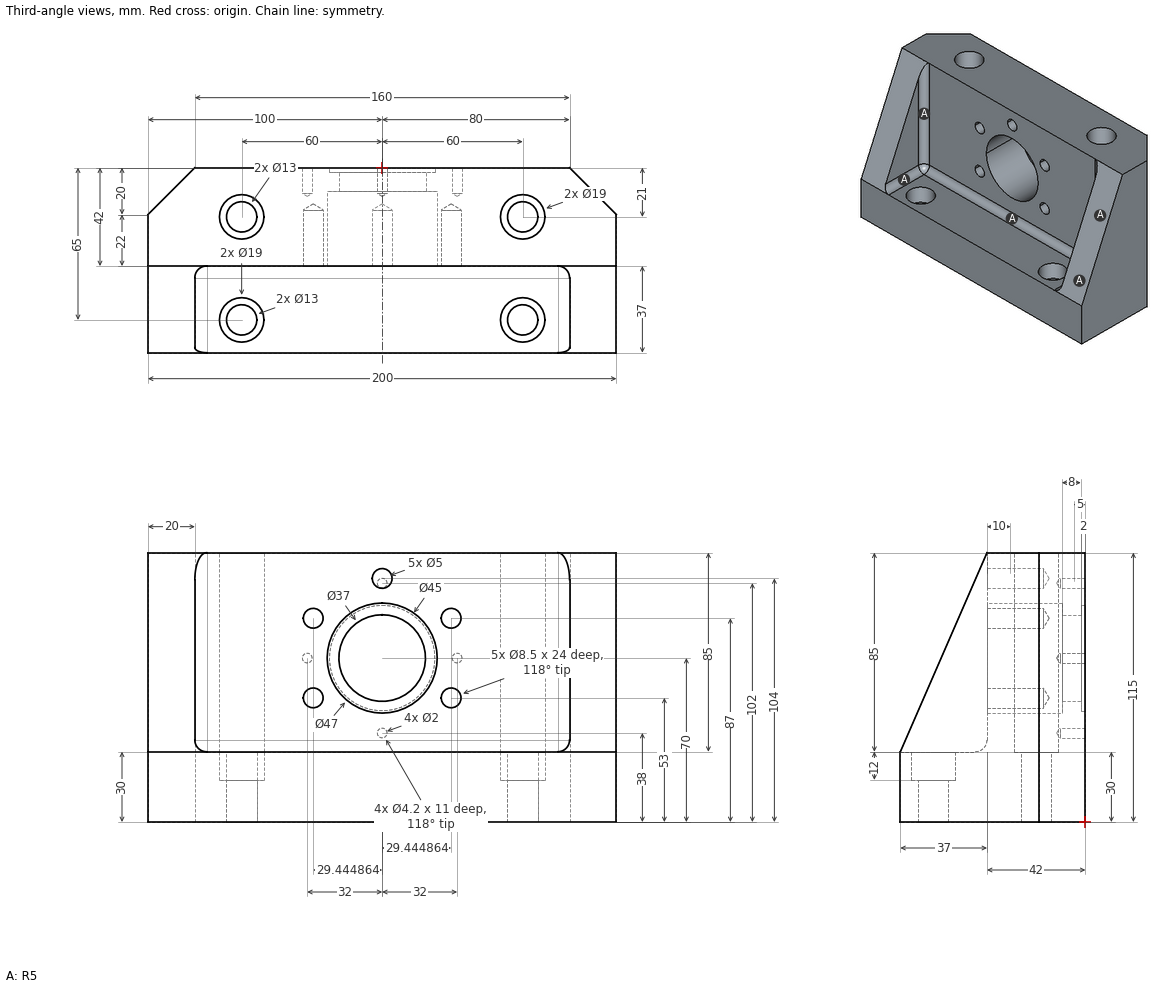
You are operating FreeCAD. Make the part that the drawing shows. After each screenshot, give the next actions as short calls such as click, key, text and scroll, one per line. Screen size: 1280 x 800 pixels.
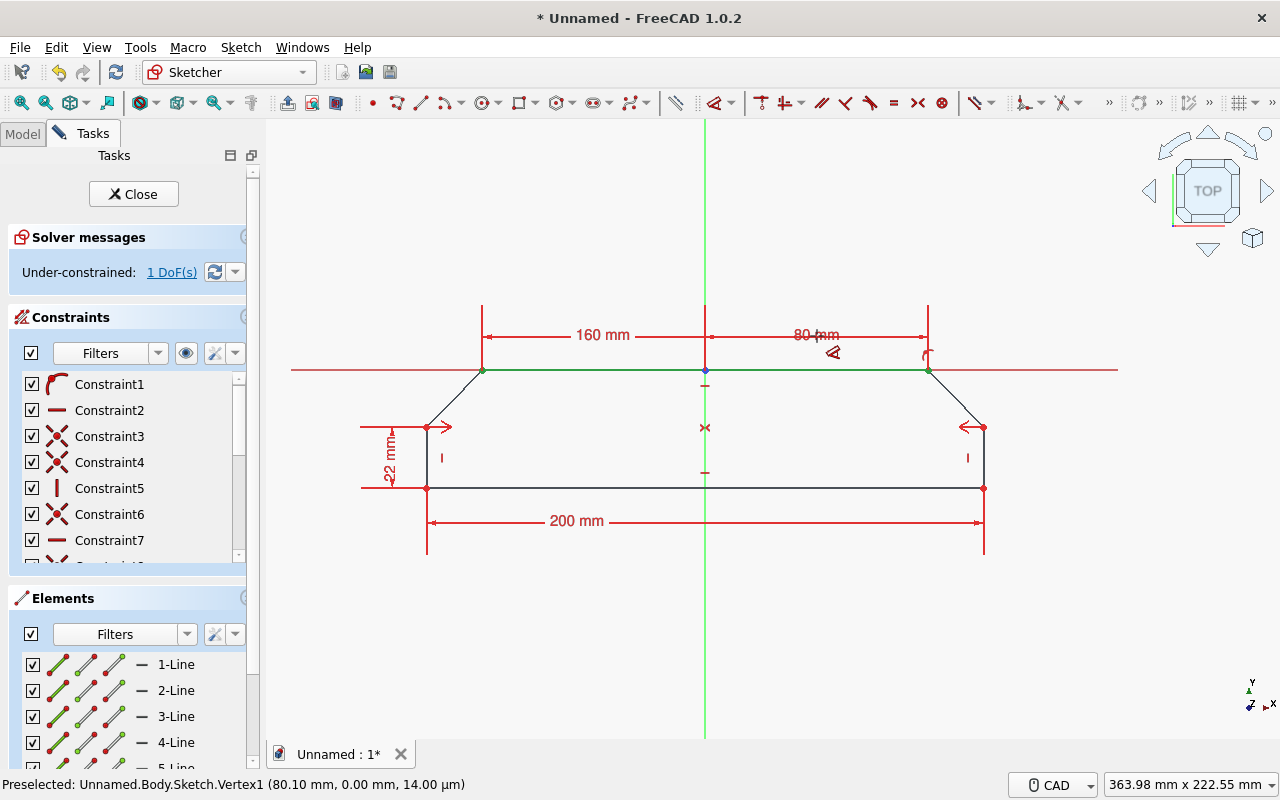
click(427, 427)
click(393, 399)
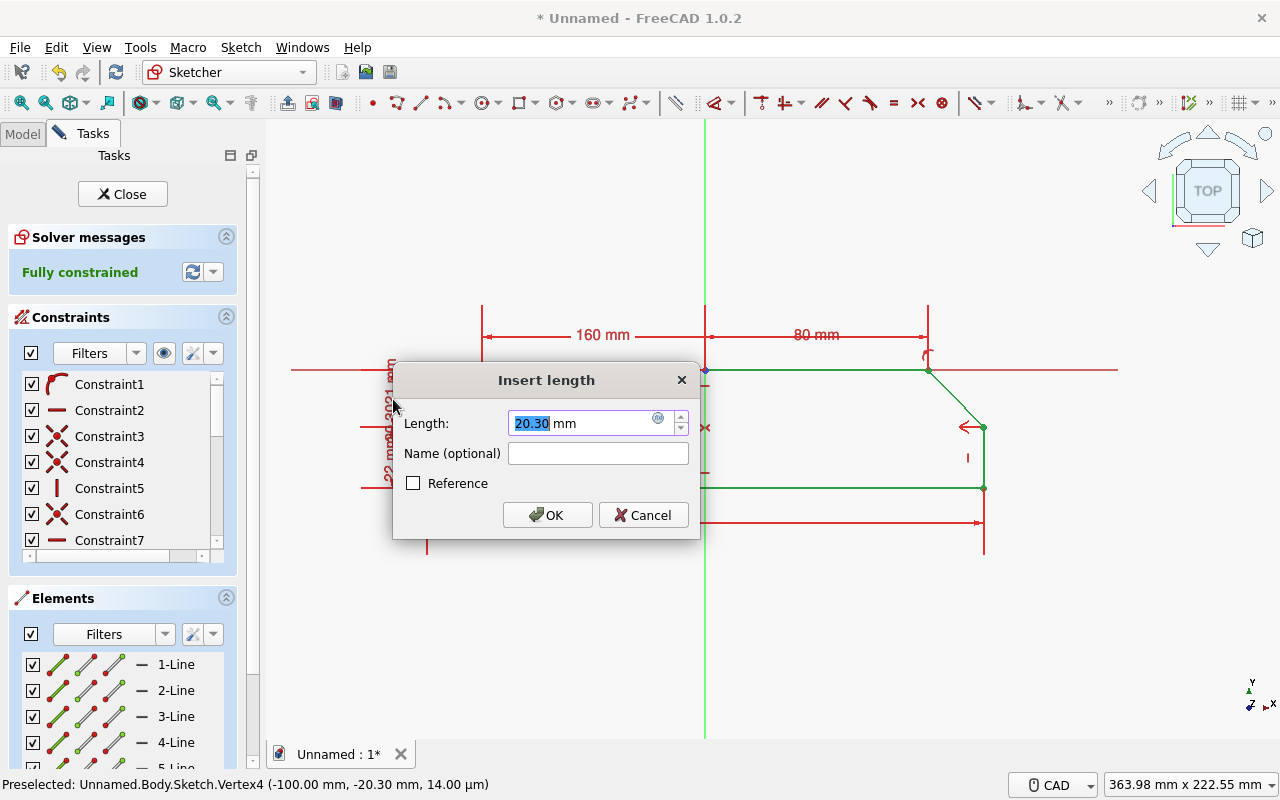
text(20)
key(Return)
key(Escape)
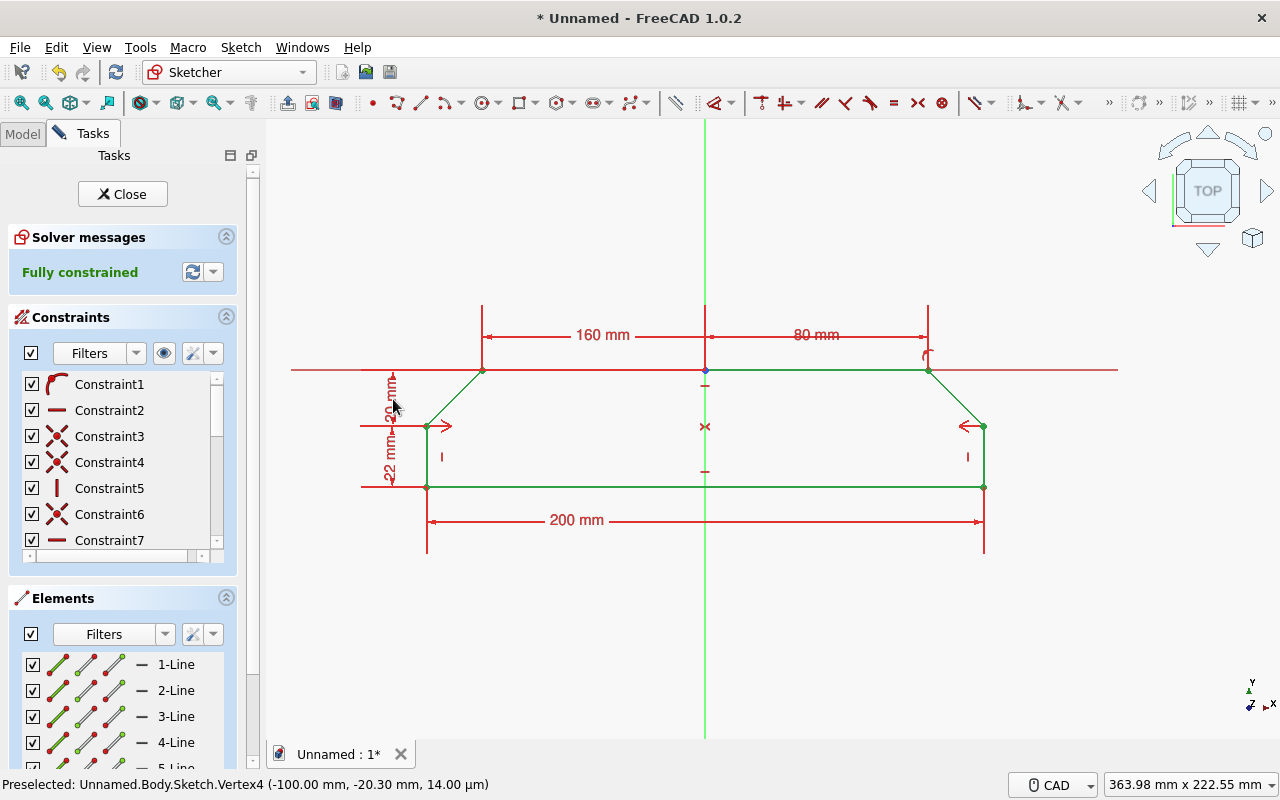
click(123, 194)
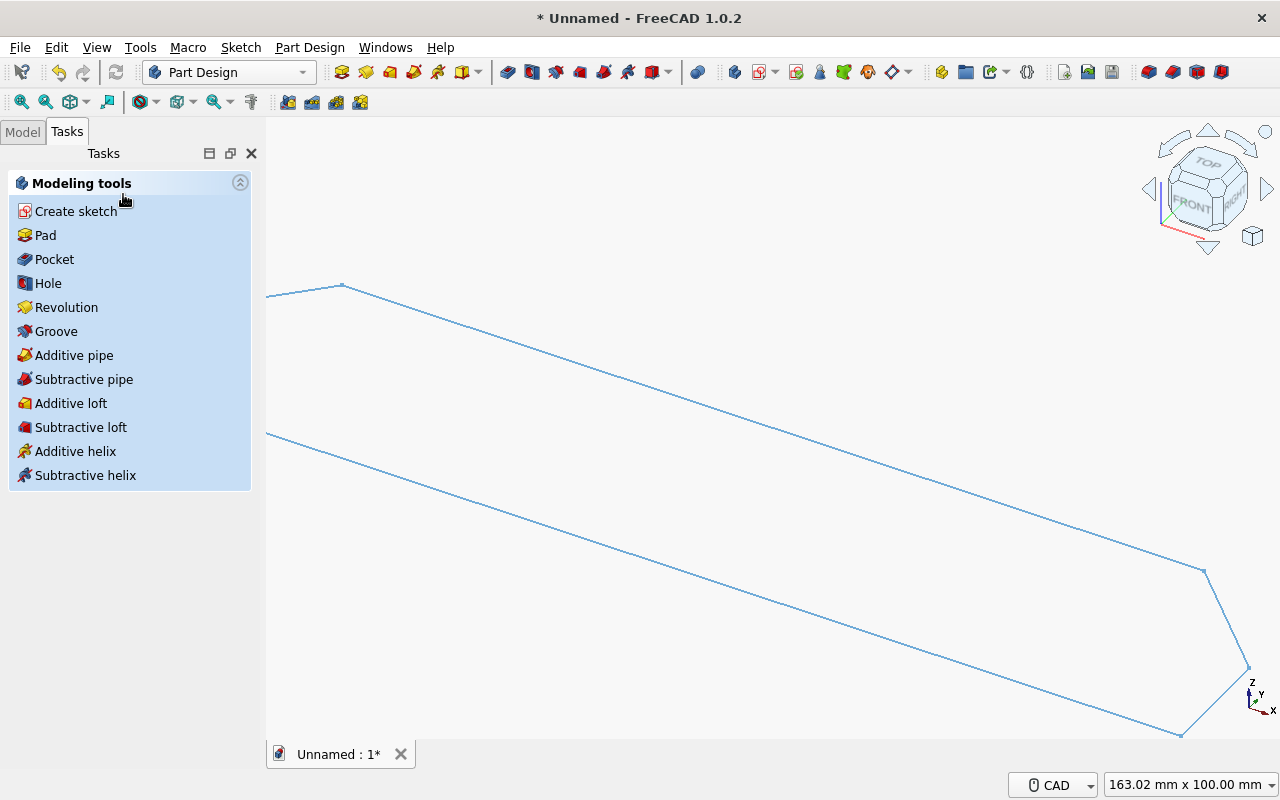
click(342, 72)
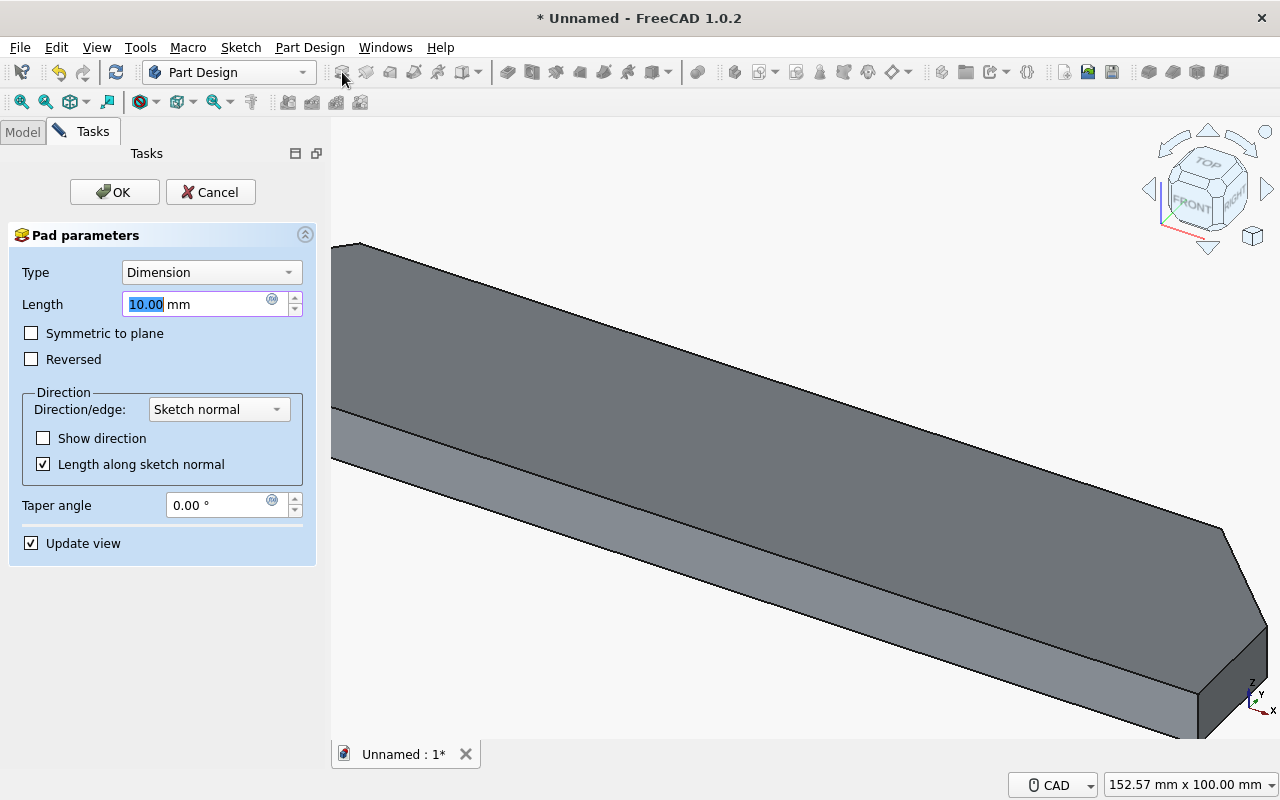
text(115)
key(Tab)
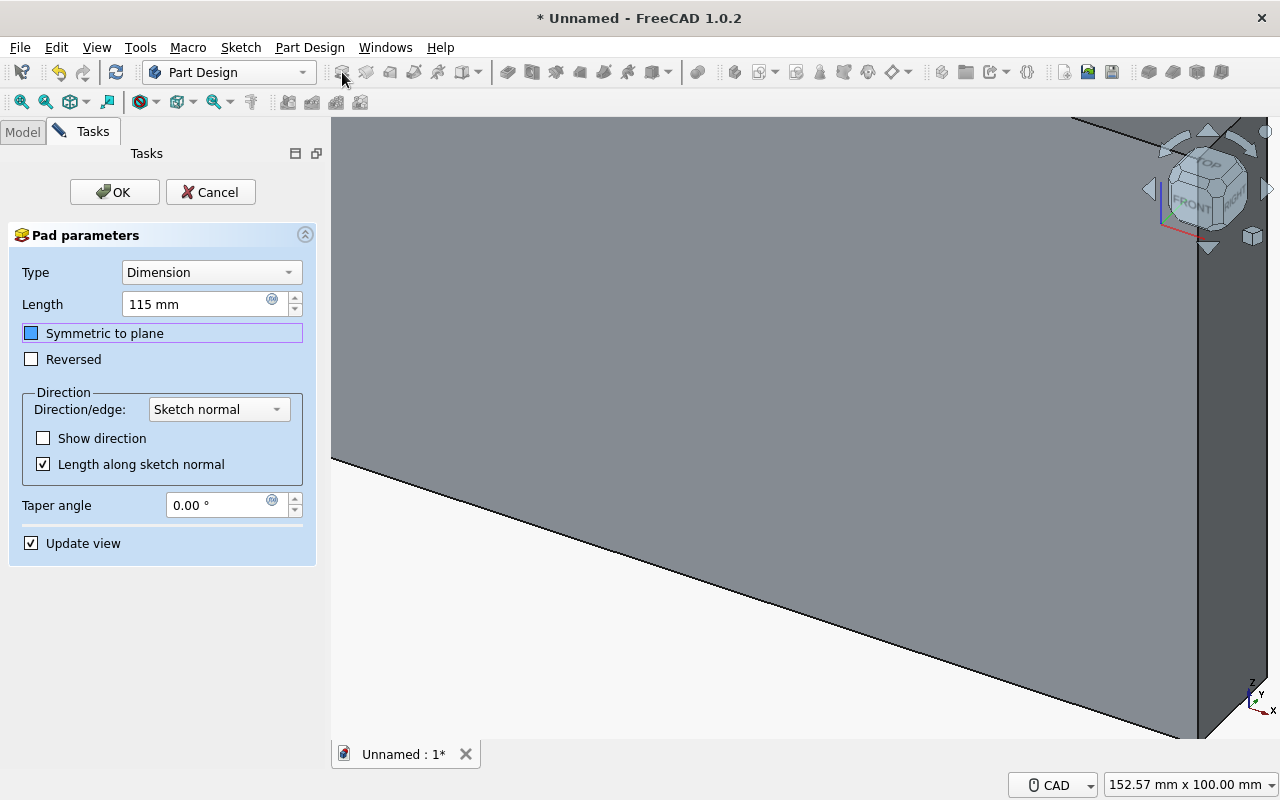
click(115, 192)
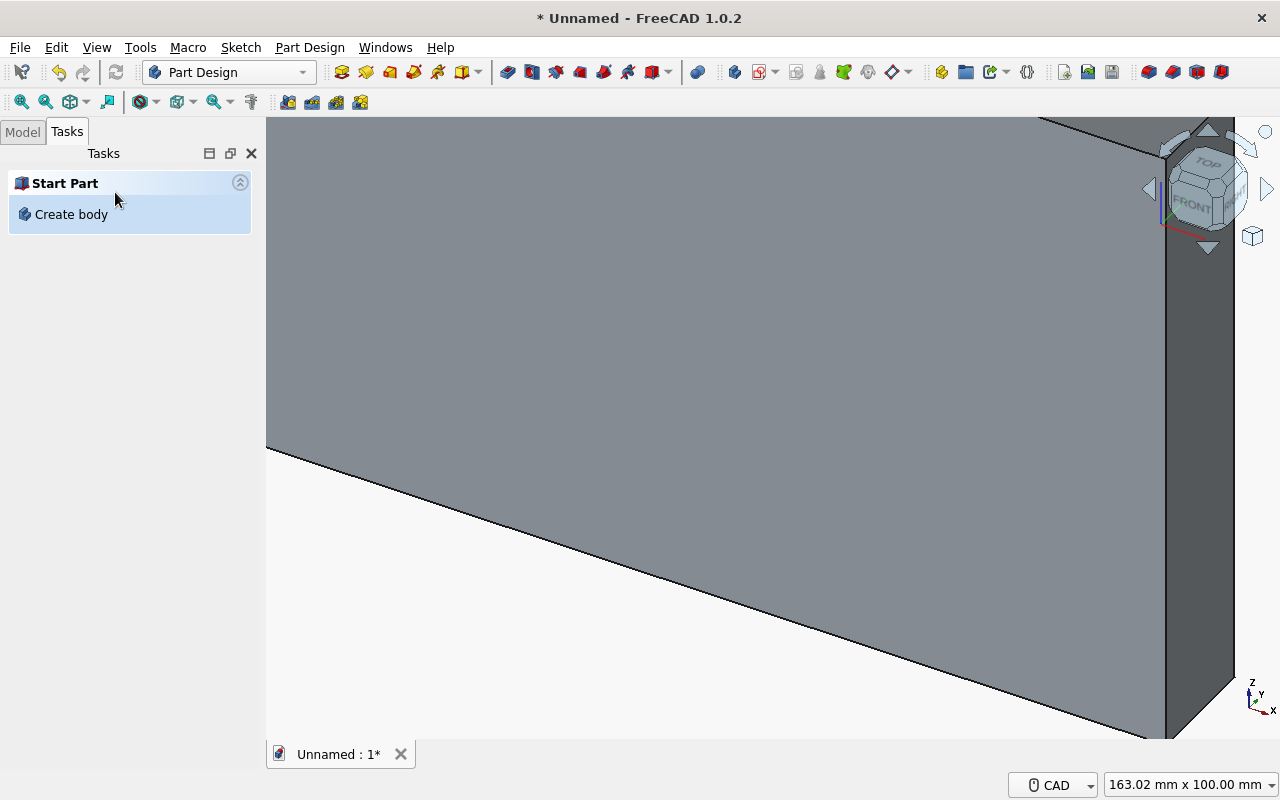
click(22, 102)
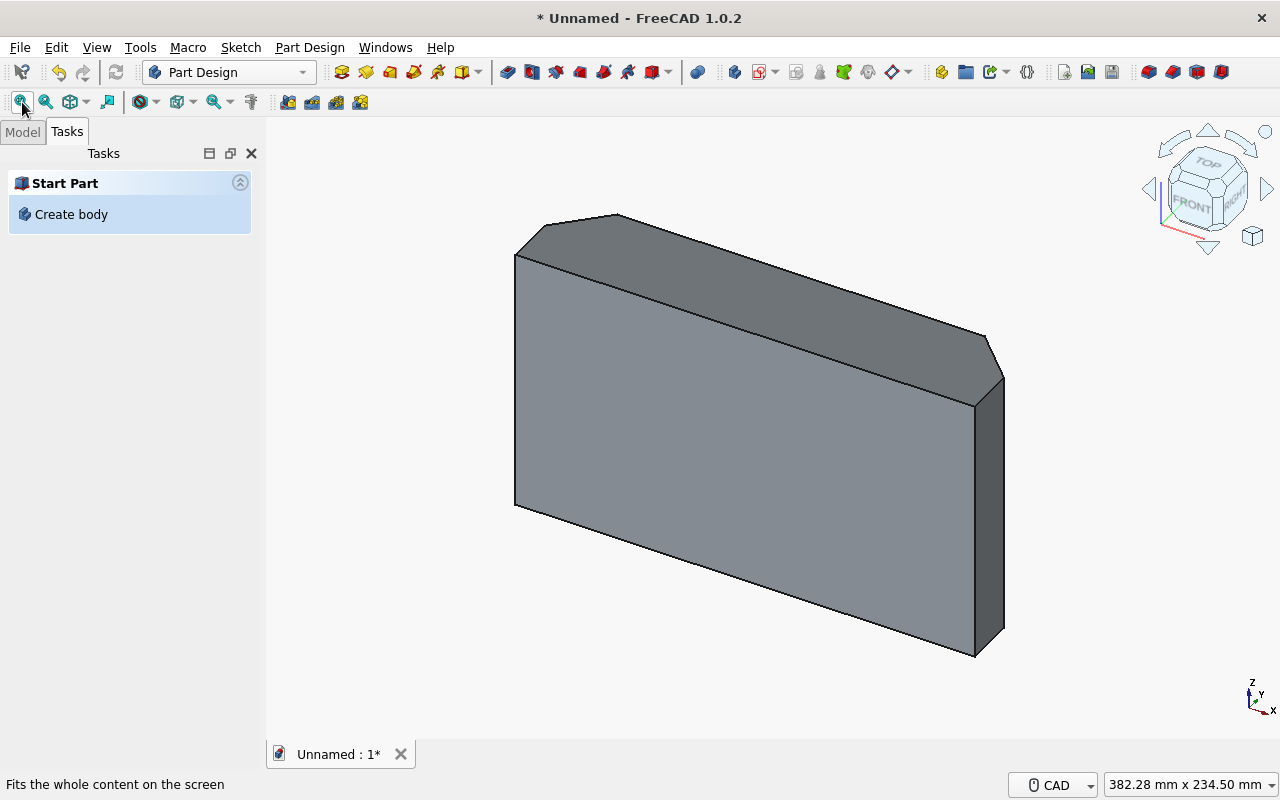
click(760, 72)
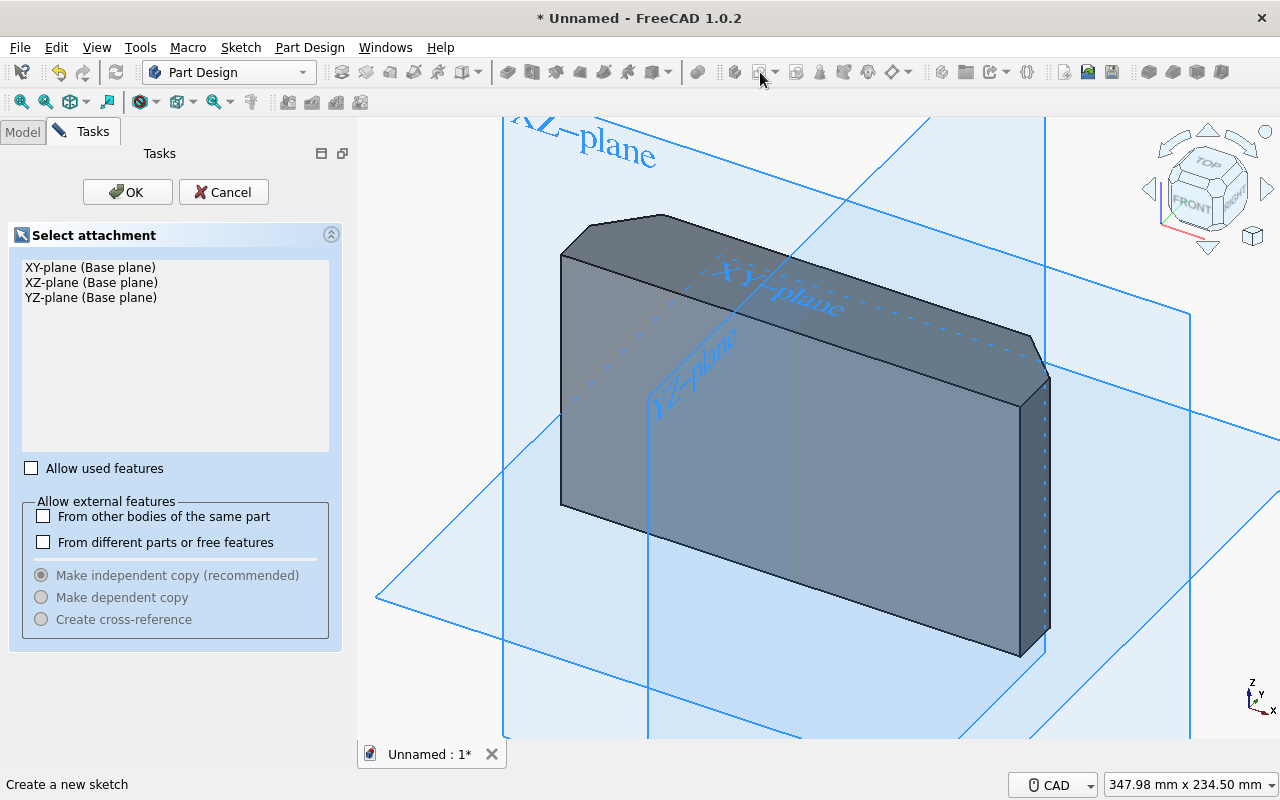
click(82, 268)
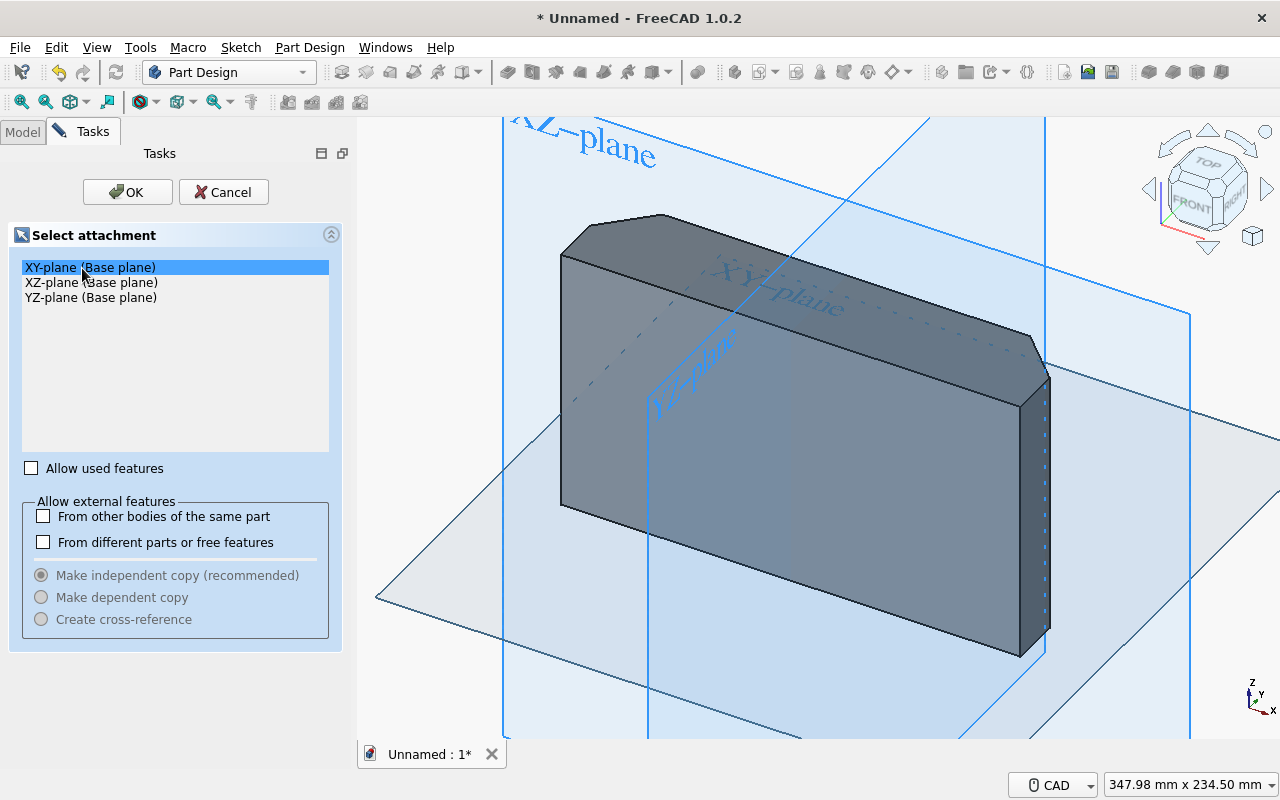
click(128, 192)